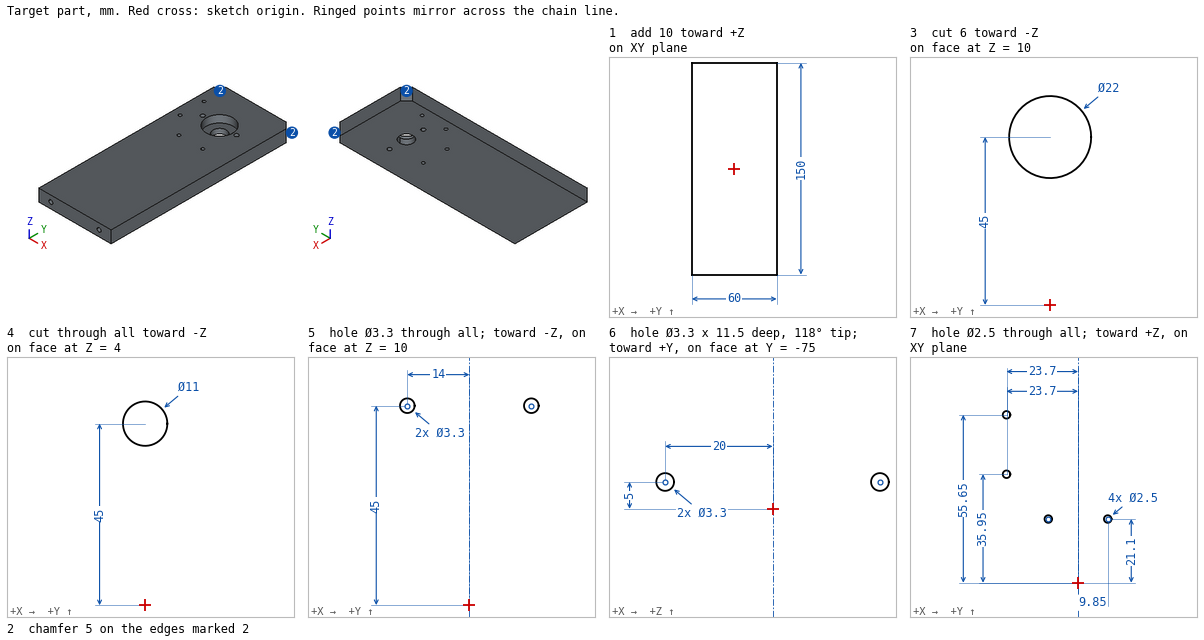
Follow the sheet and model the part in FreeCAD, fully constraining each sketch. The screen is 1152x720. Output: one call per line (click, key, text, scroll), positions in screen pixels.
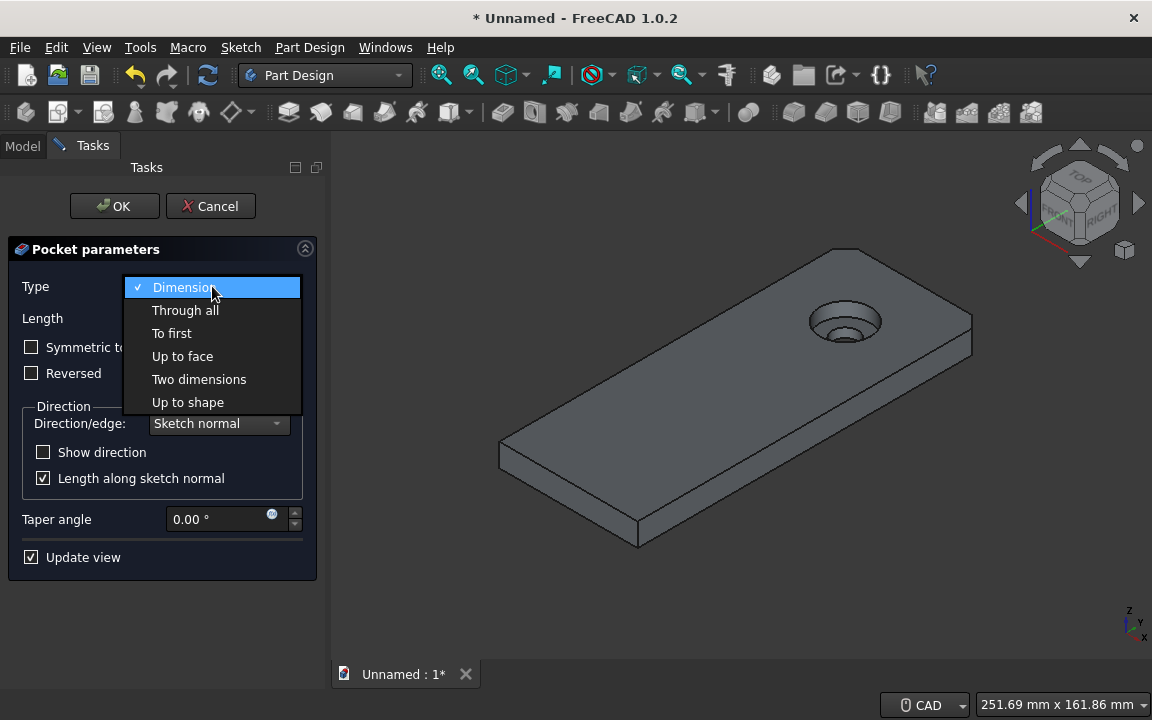
click(212, 310)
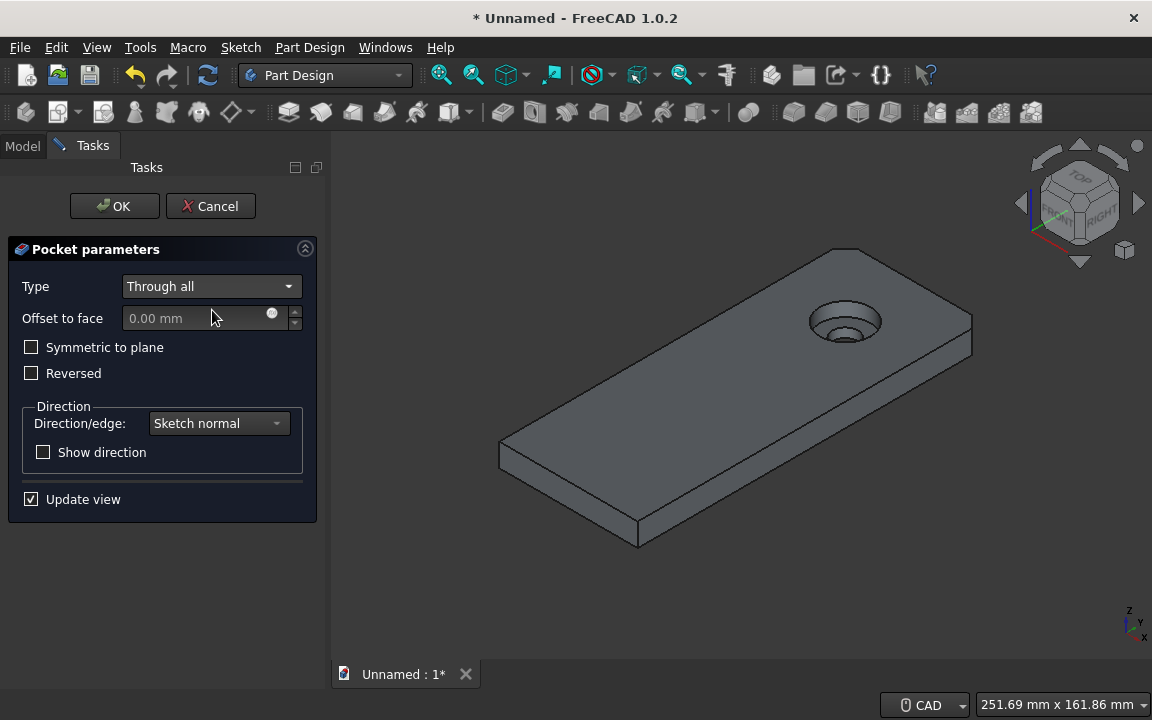
click(115, 206)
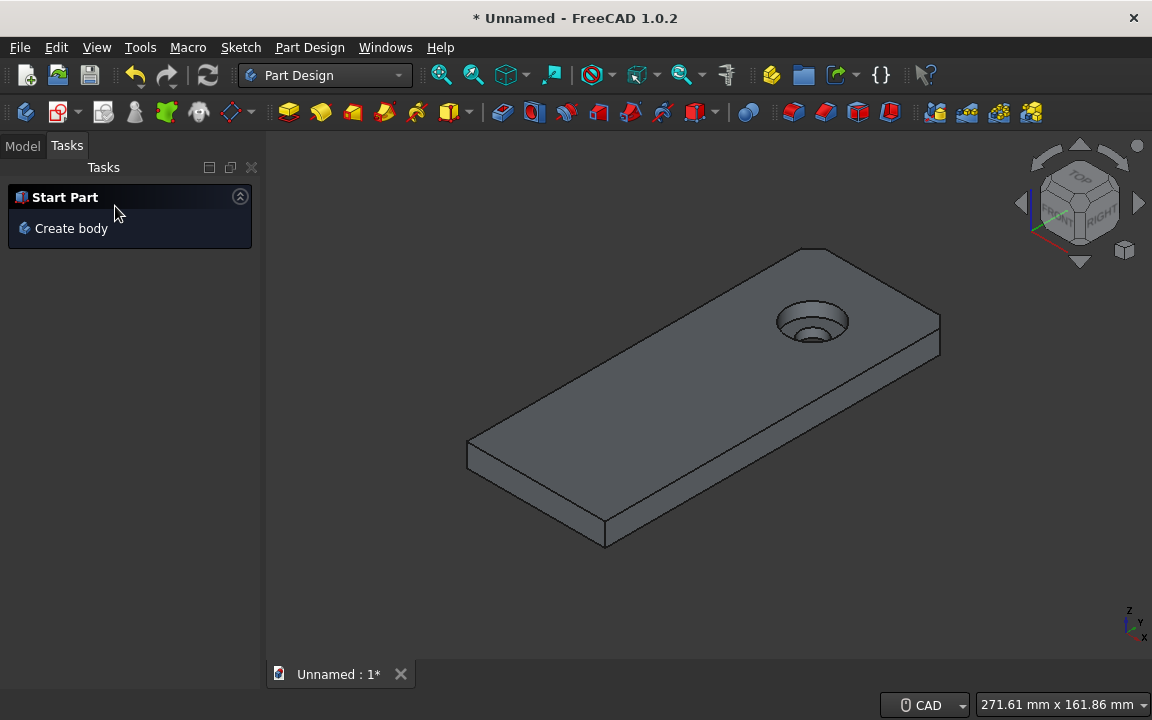
click(709, 381)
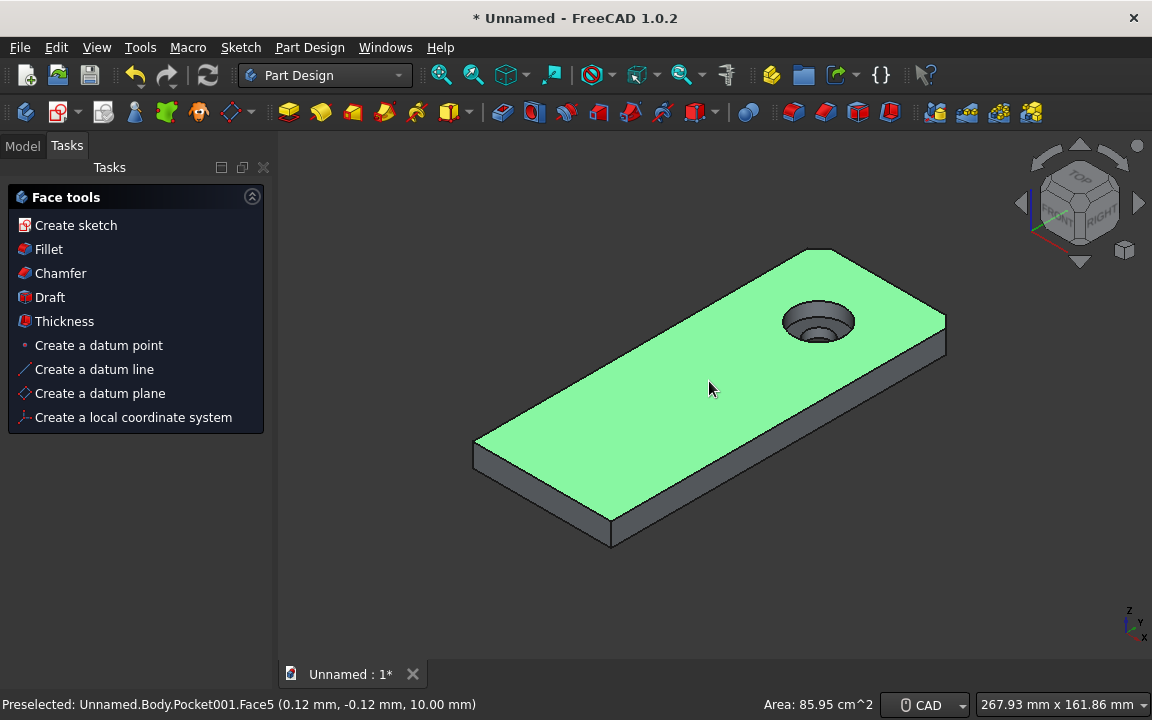
click(58, 112)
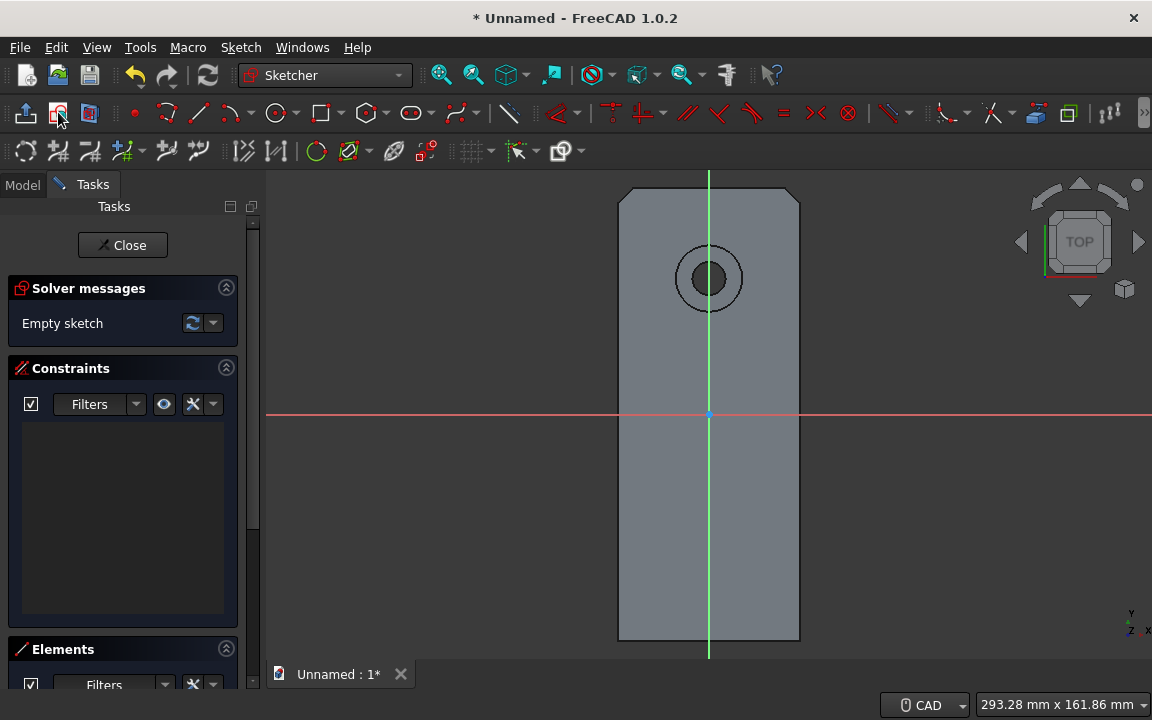
scroll(765, 287, up, 4)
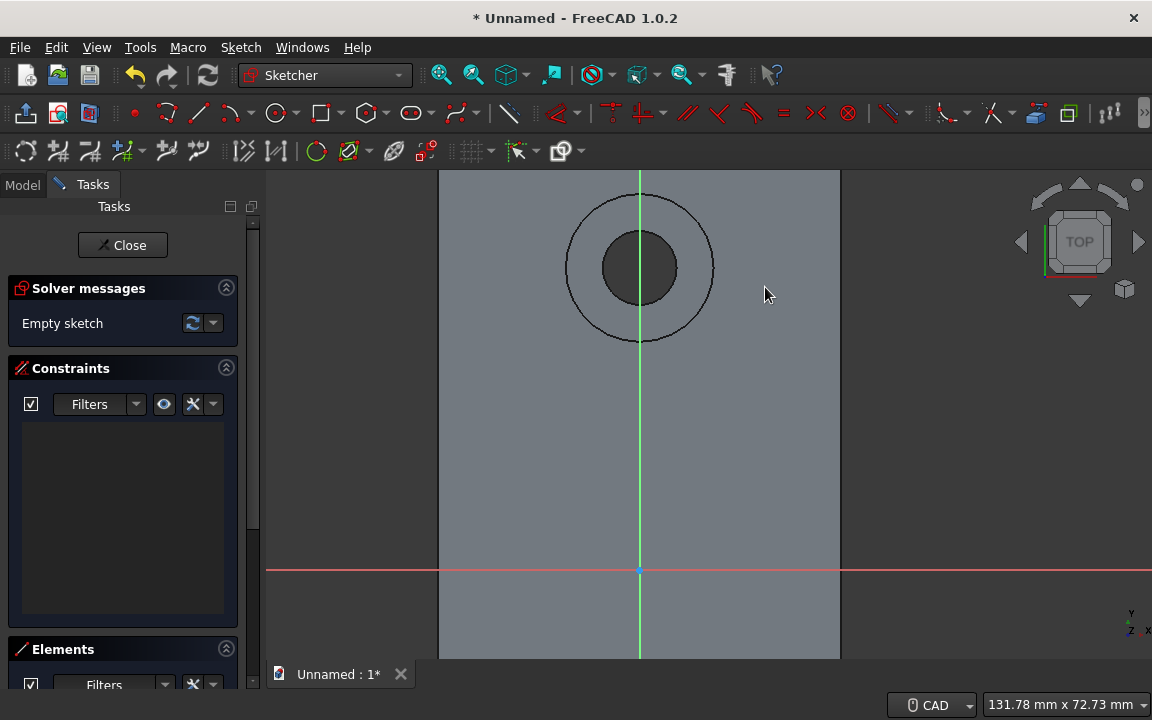
click(276, 114)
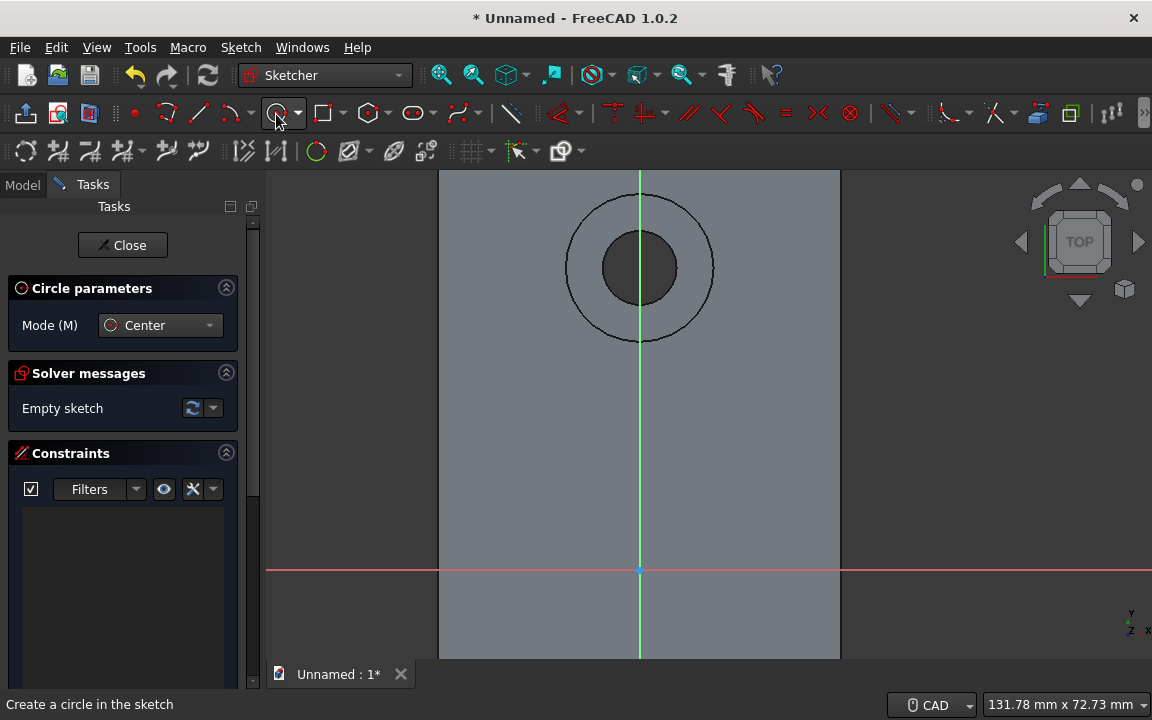
scroll(546, 268, up, 4)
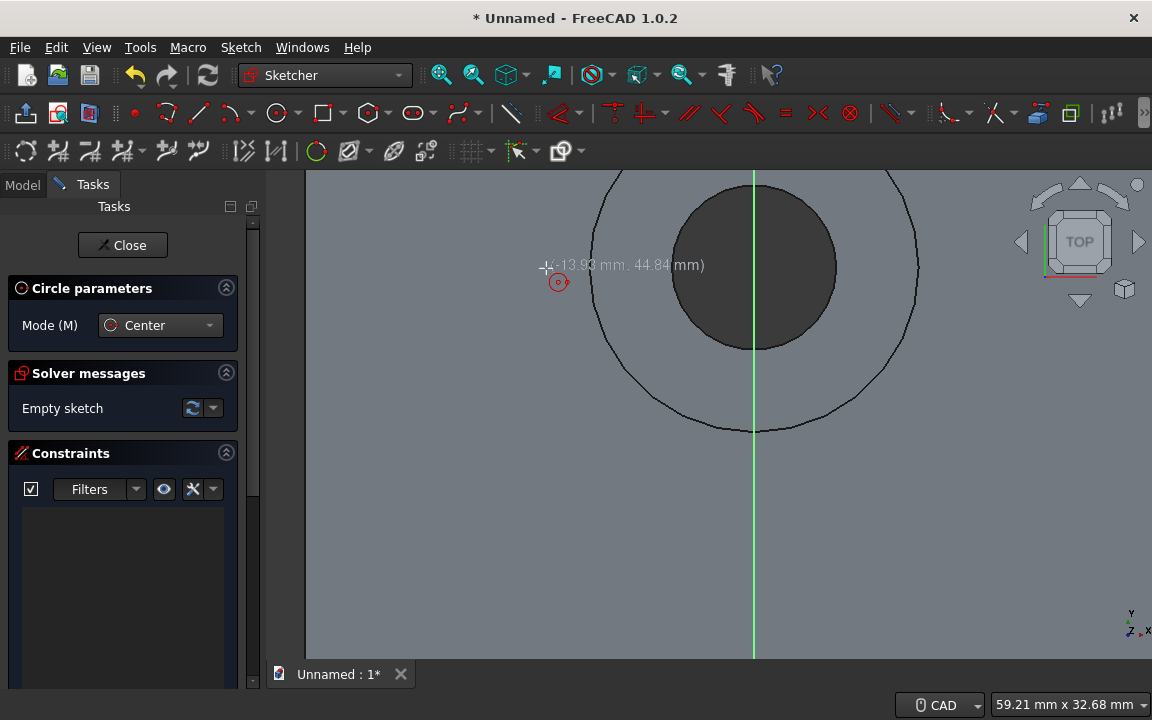
click(545, 268)
click(562, 250)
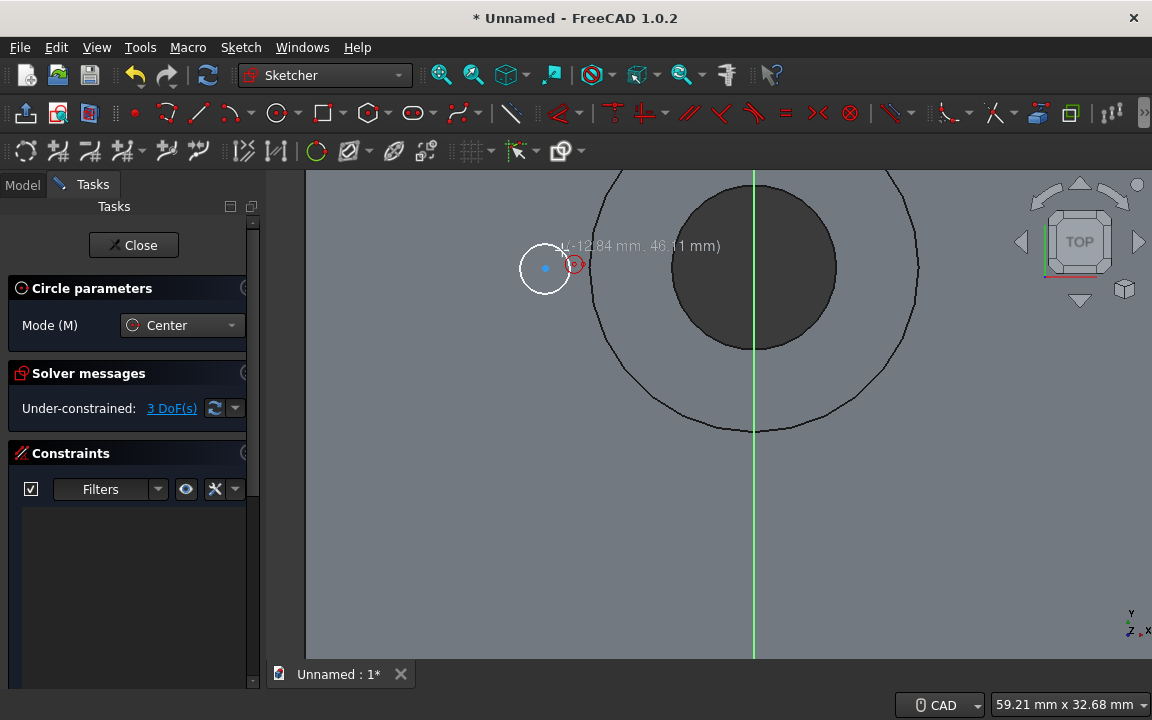
click(964, 268)
click(981, 250)
key(Escape)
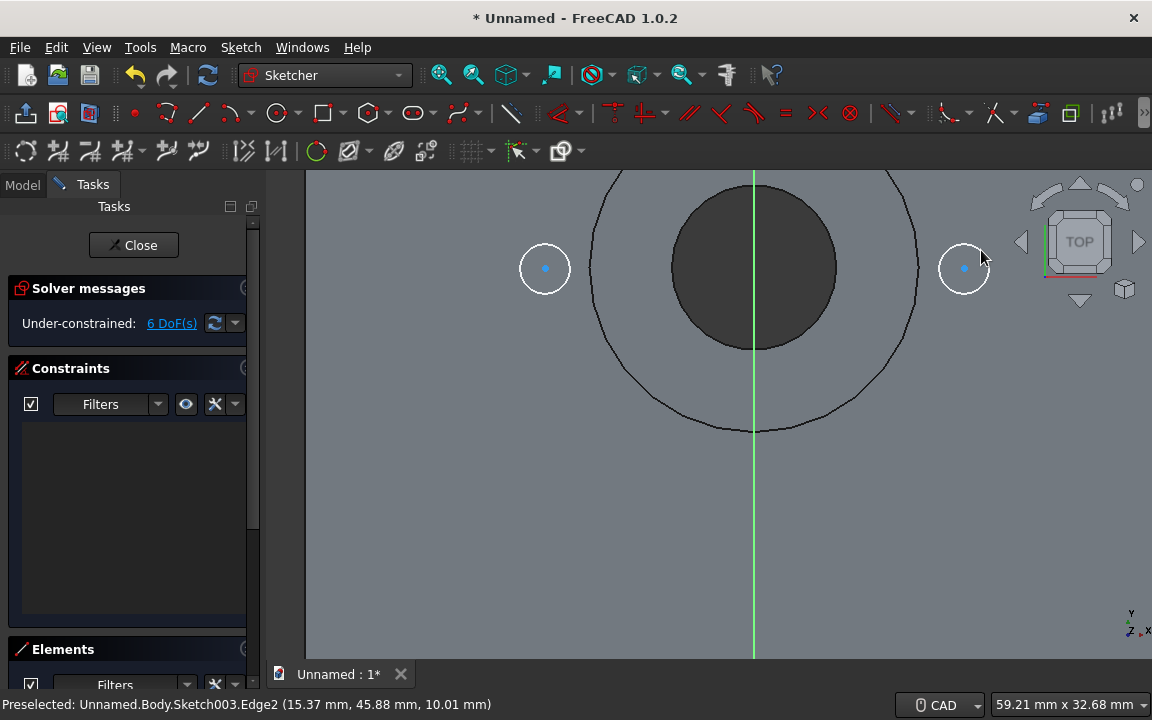
click(562, 251)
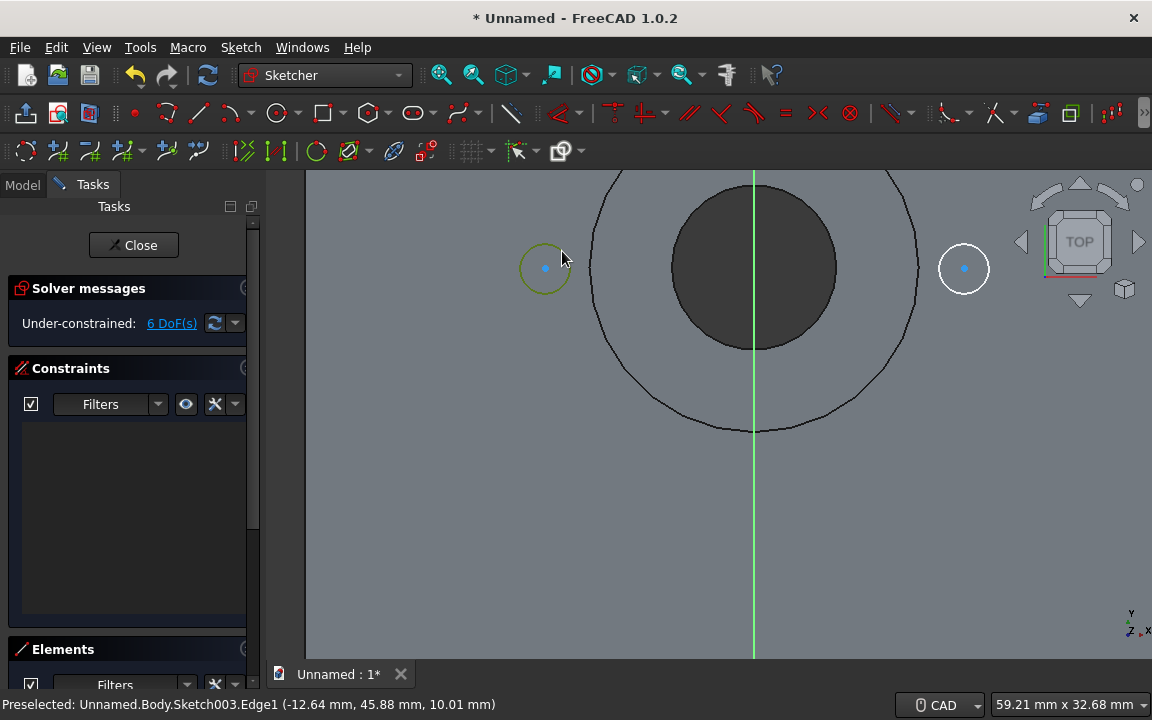
click(981, 251)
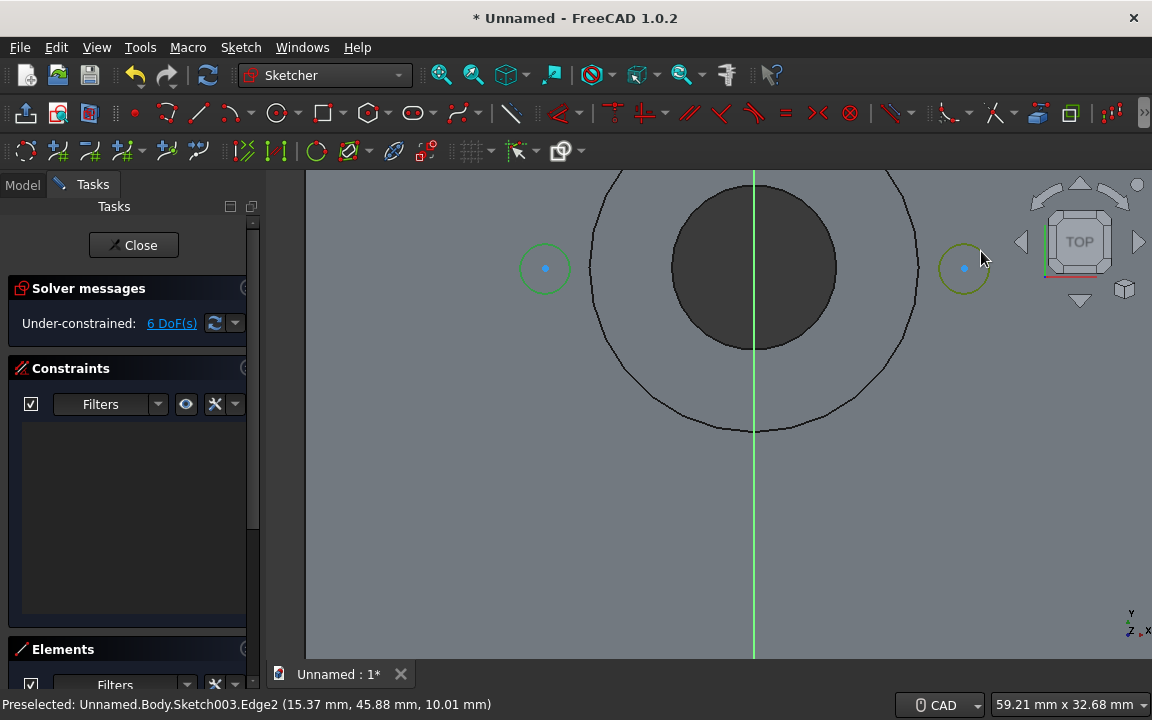
click(786, 114)